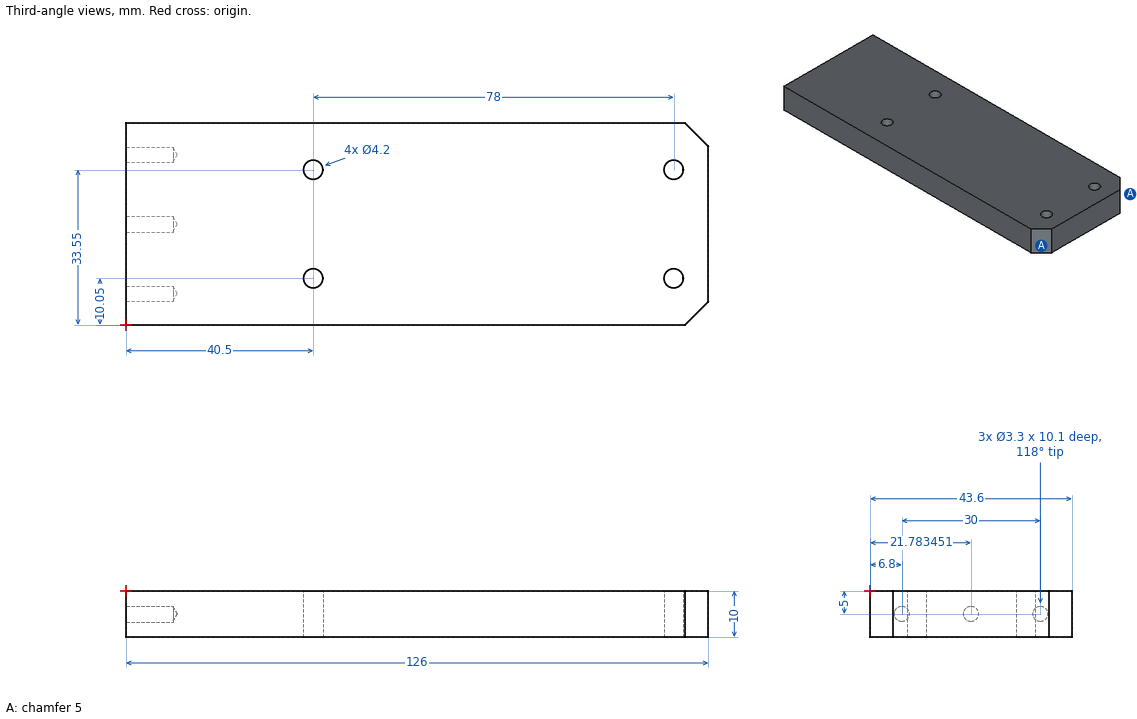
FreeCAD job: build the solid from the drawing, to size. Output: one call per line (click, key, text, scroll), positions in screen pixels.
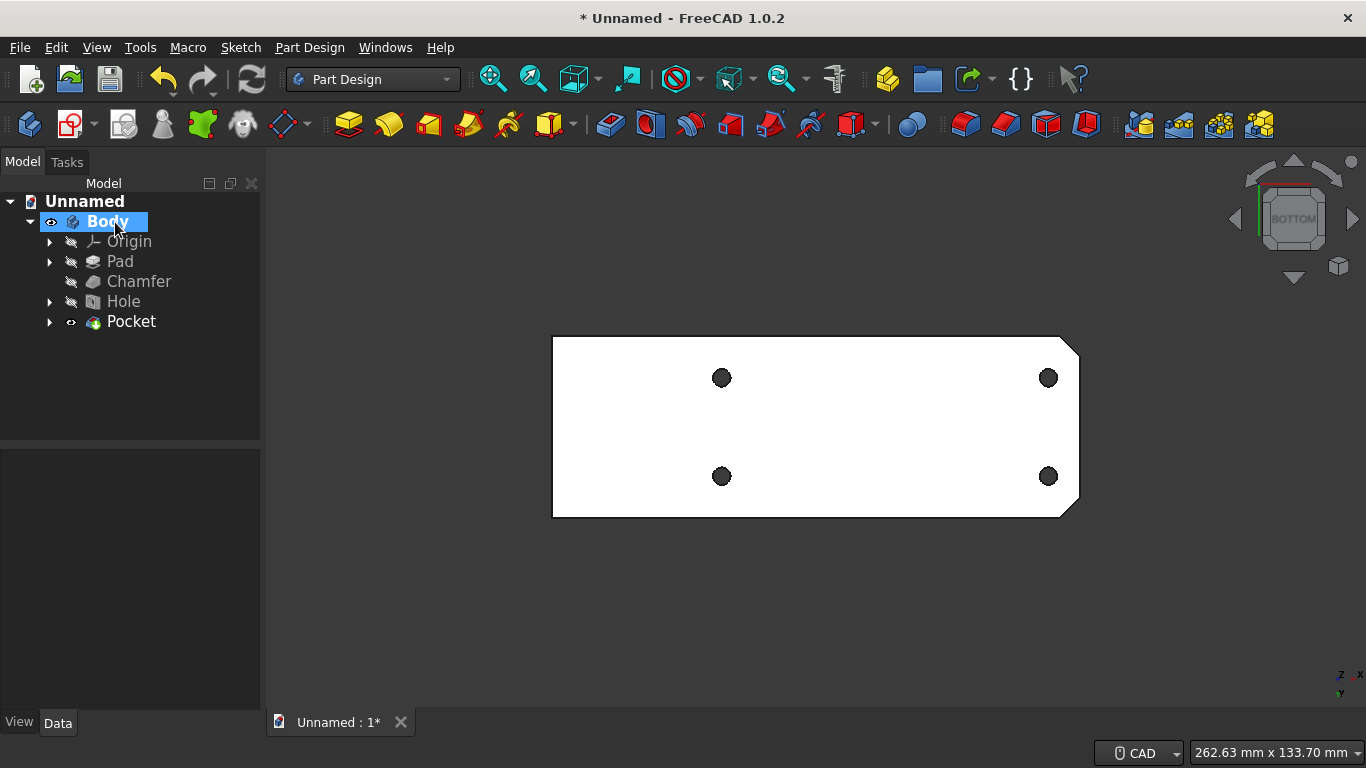
key(0)